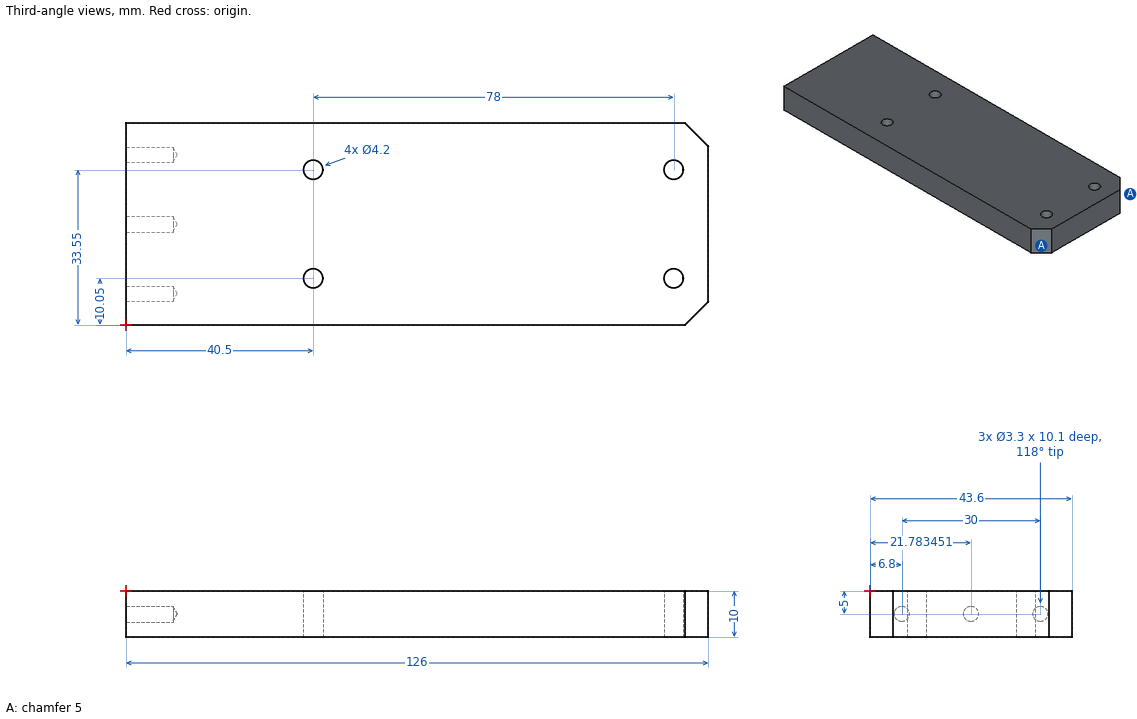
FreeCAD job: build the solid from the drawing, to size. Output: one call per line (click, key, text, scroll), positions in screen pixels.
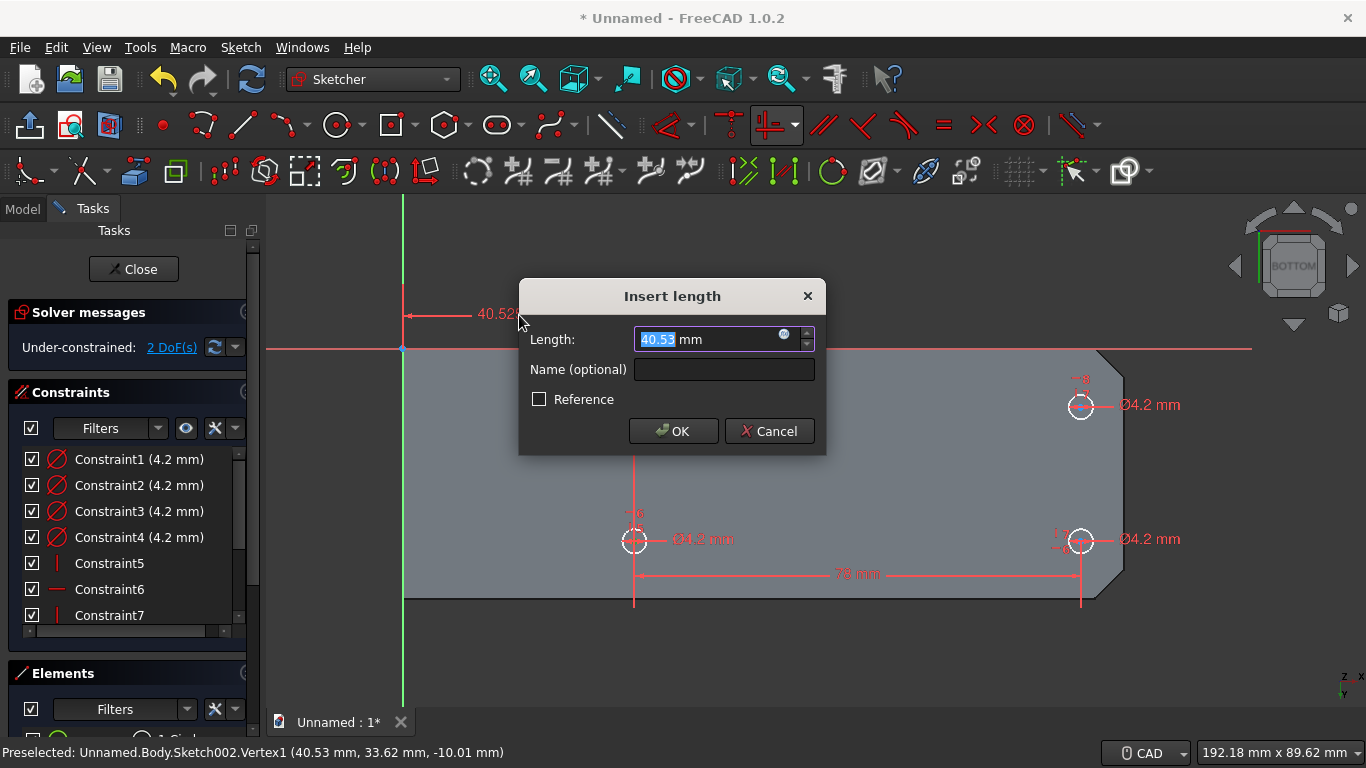
text(40.5)
key(Return)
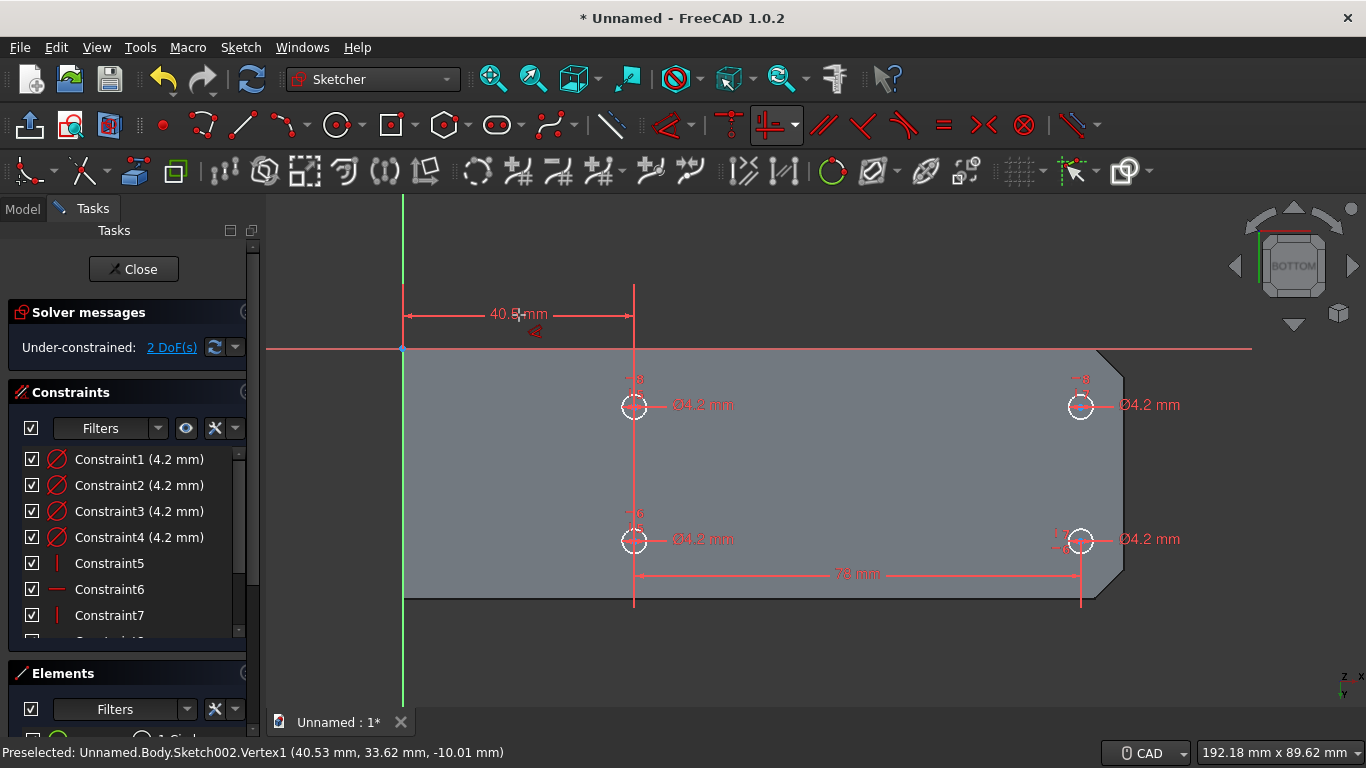
click(634, 541)
click(369, 445)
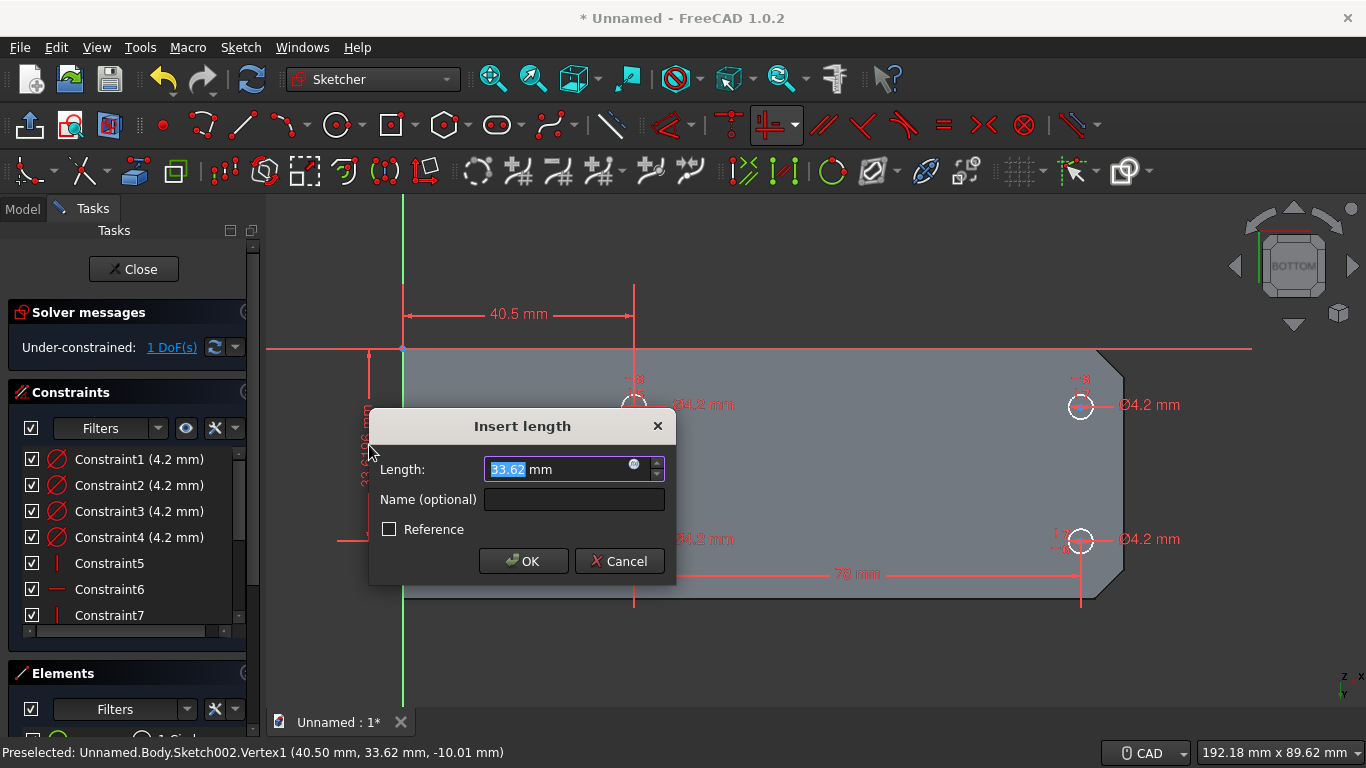
text(33.55)
key(Return)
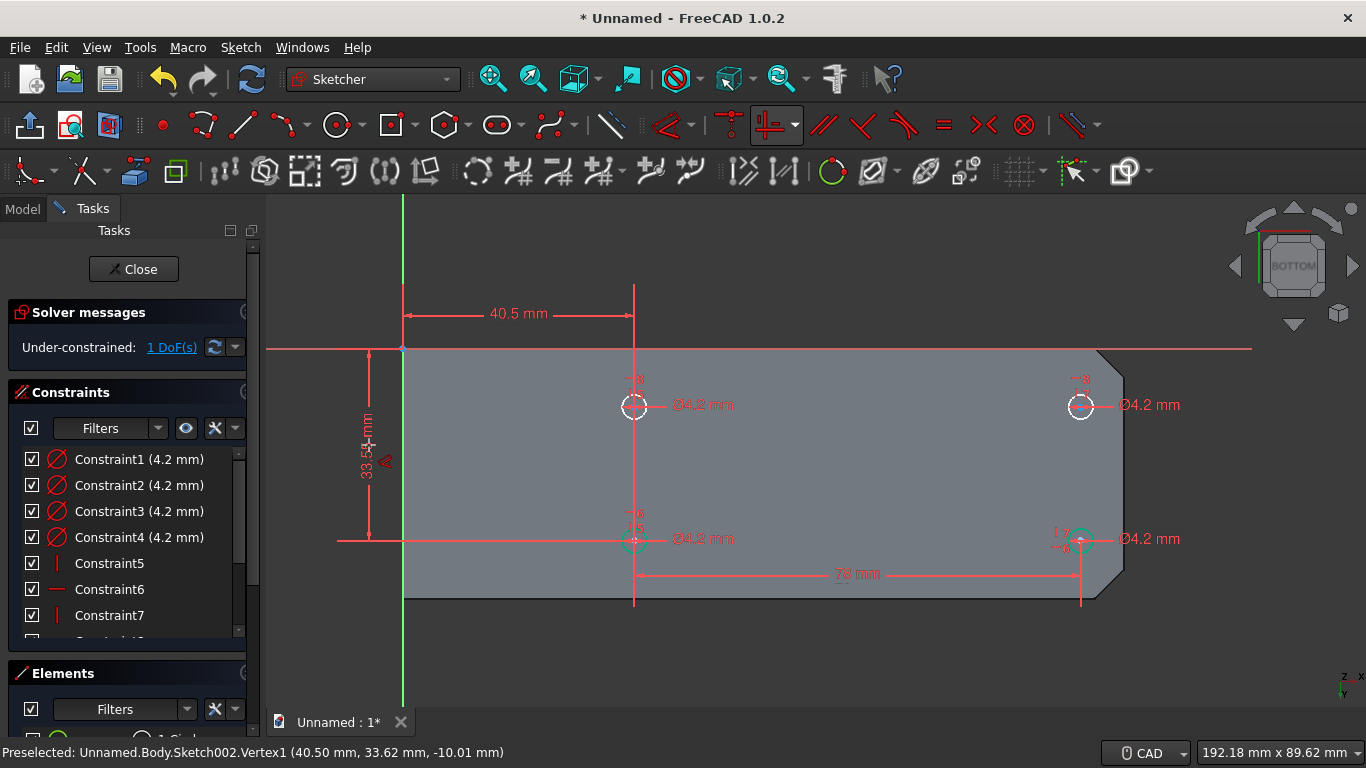
click(634, 407)
click(369, 378)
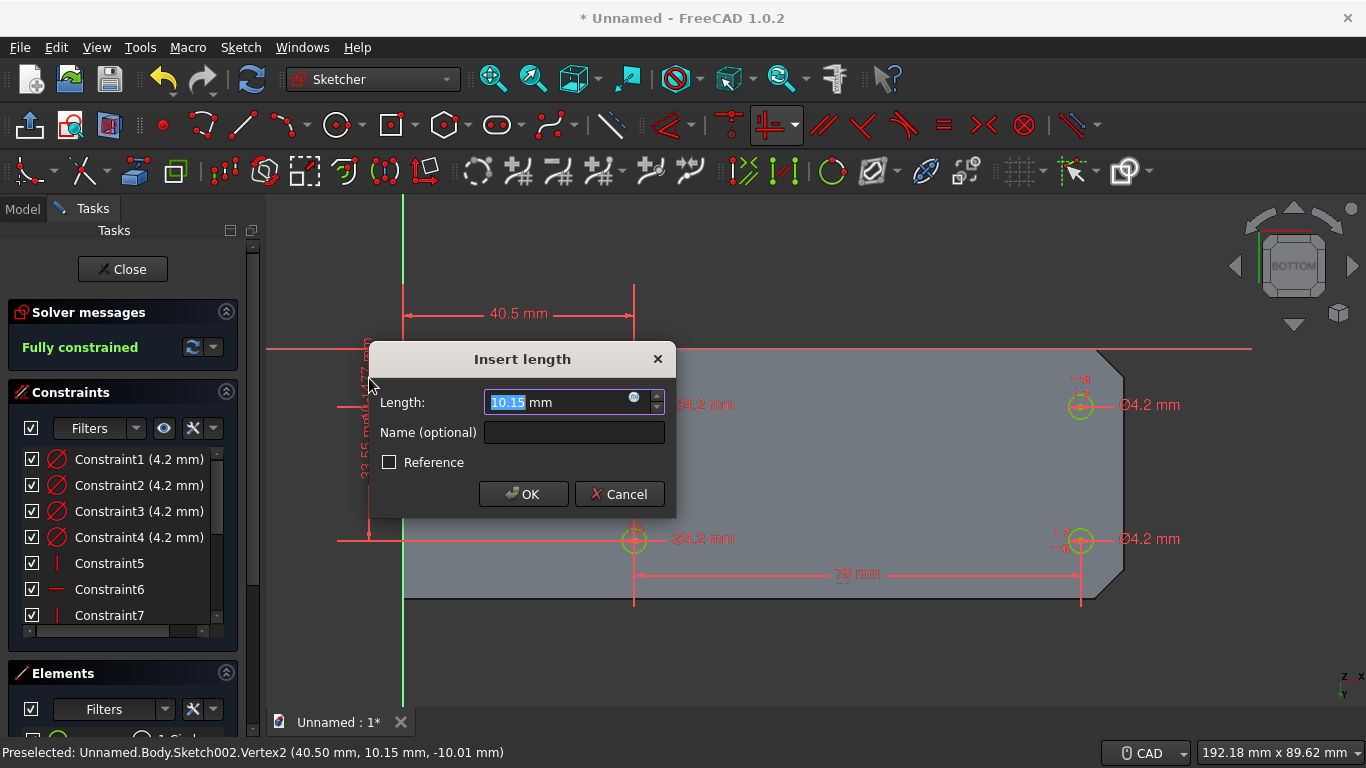
text(10.05)
key(Return)
key(Escape)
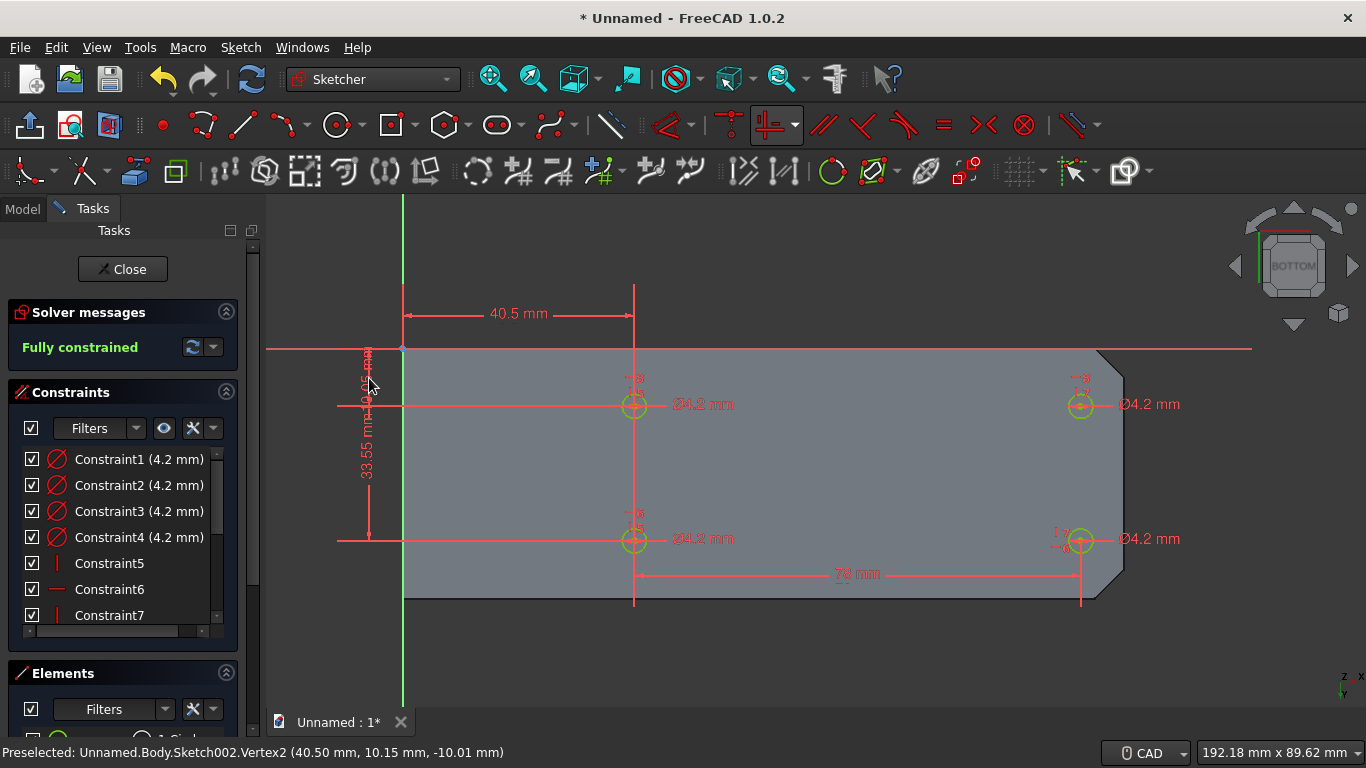
click(123, 269)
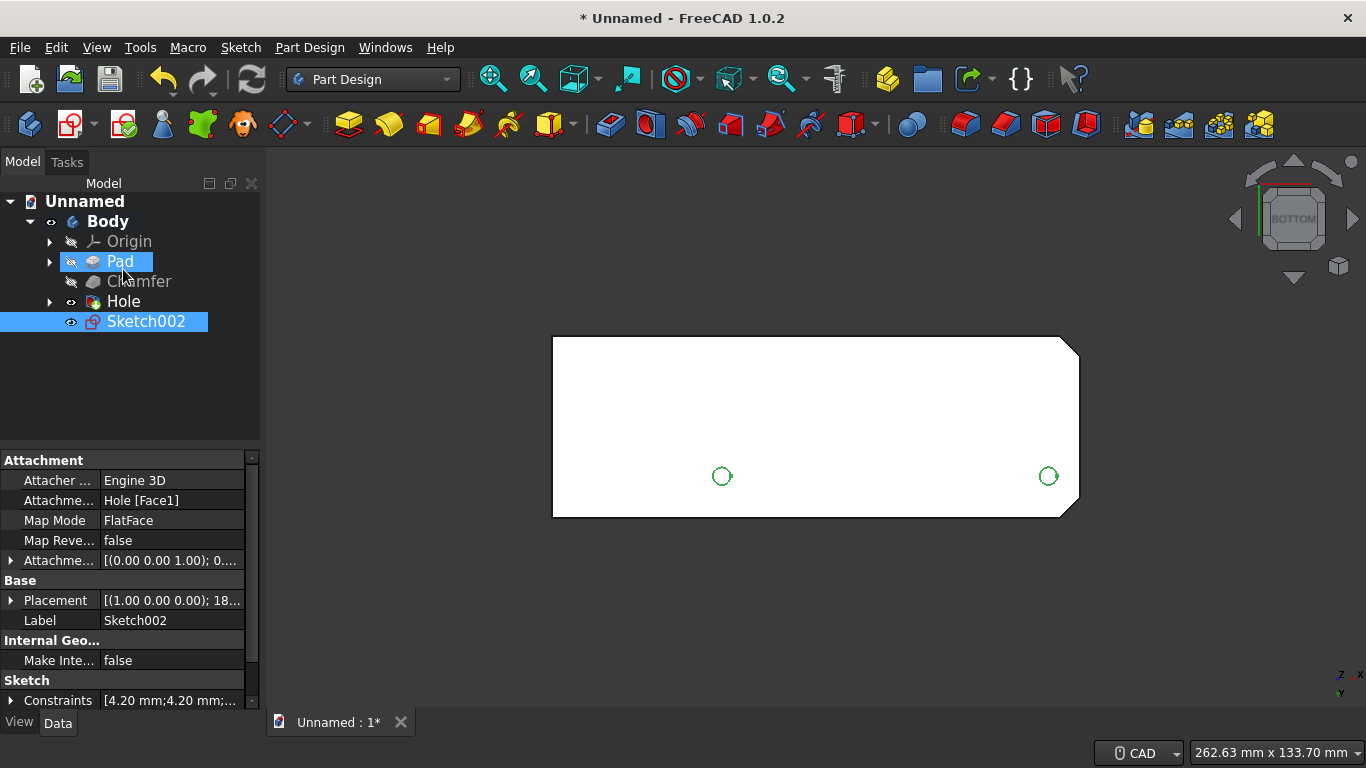
click(612, 124)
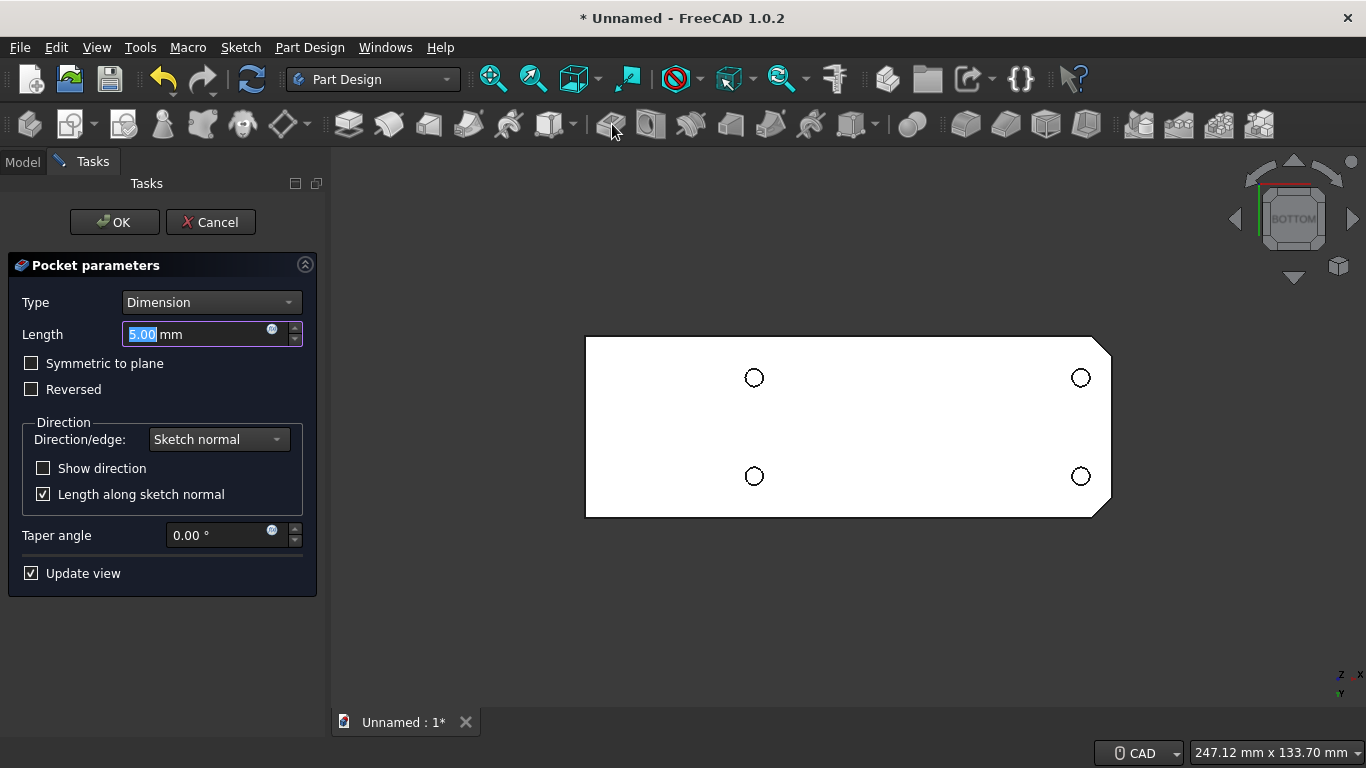
click(212, 302)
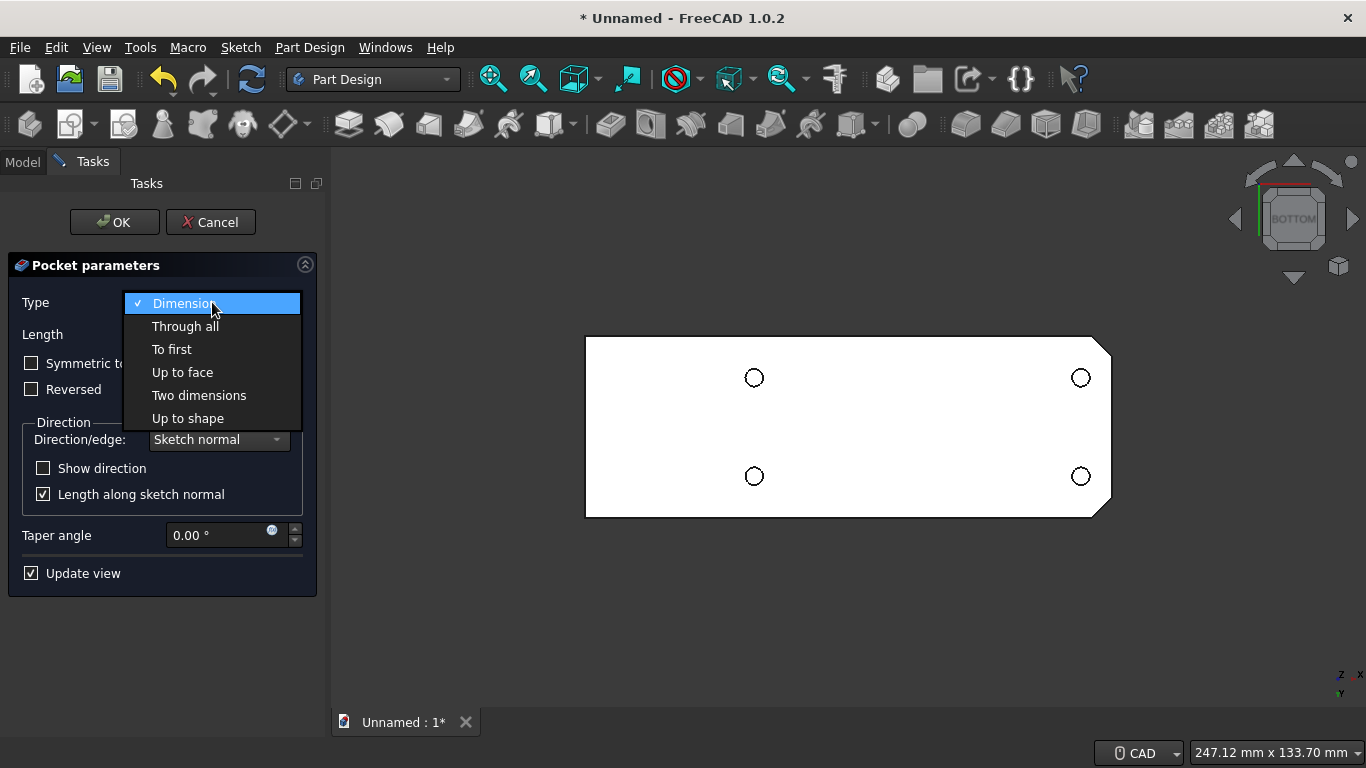
click(212, 326)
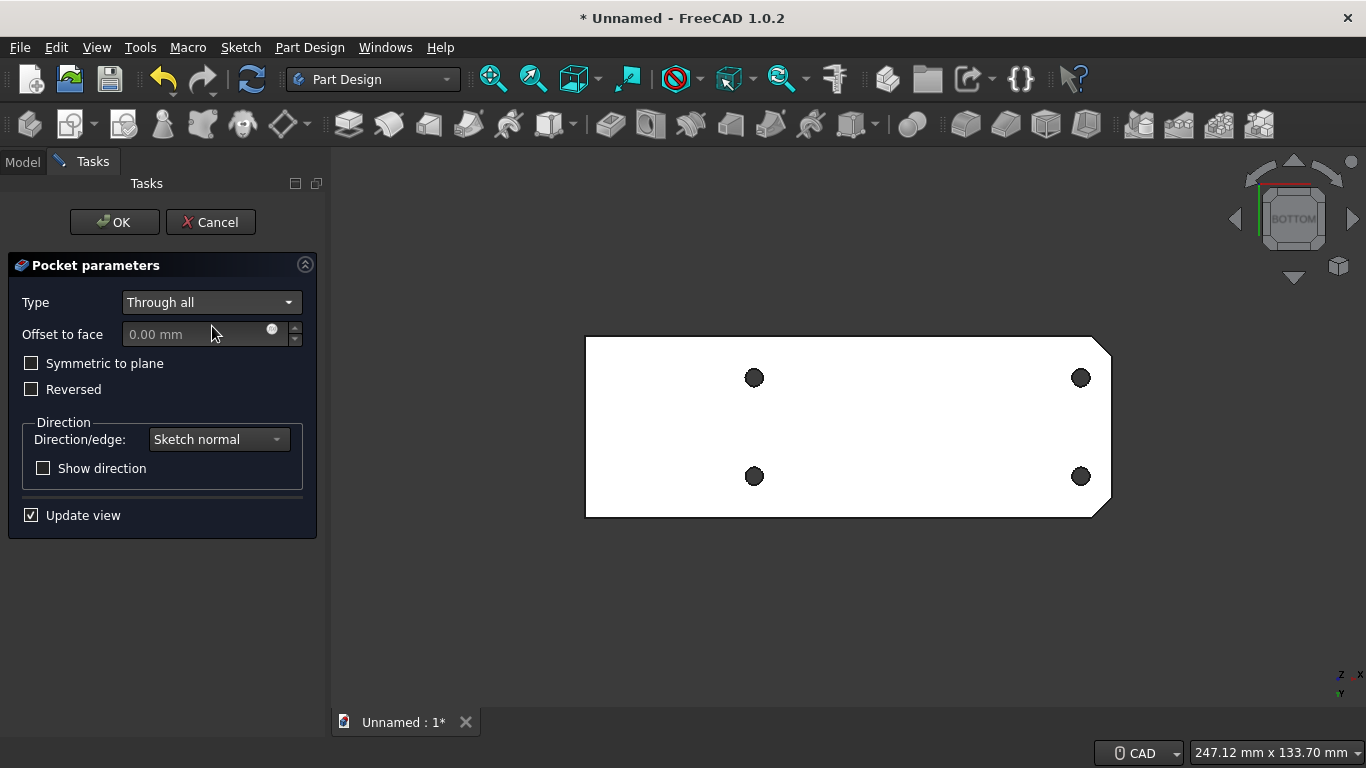
click(115, 222)